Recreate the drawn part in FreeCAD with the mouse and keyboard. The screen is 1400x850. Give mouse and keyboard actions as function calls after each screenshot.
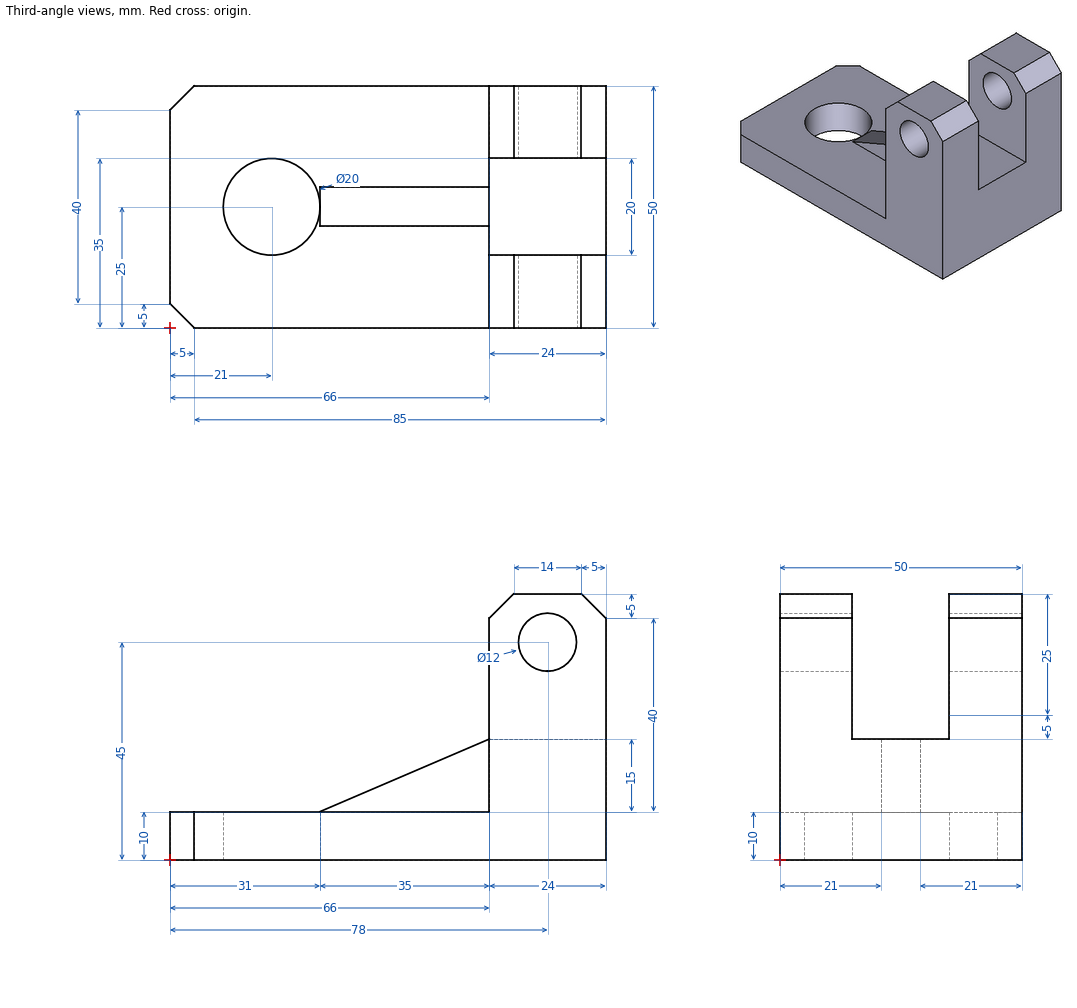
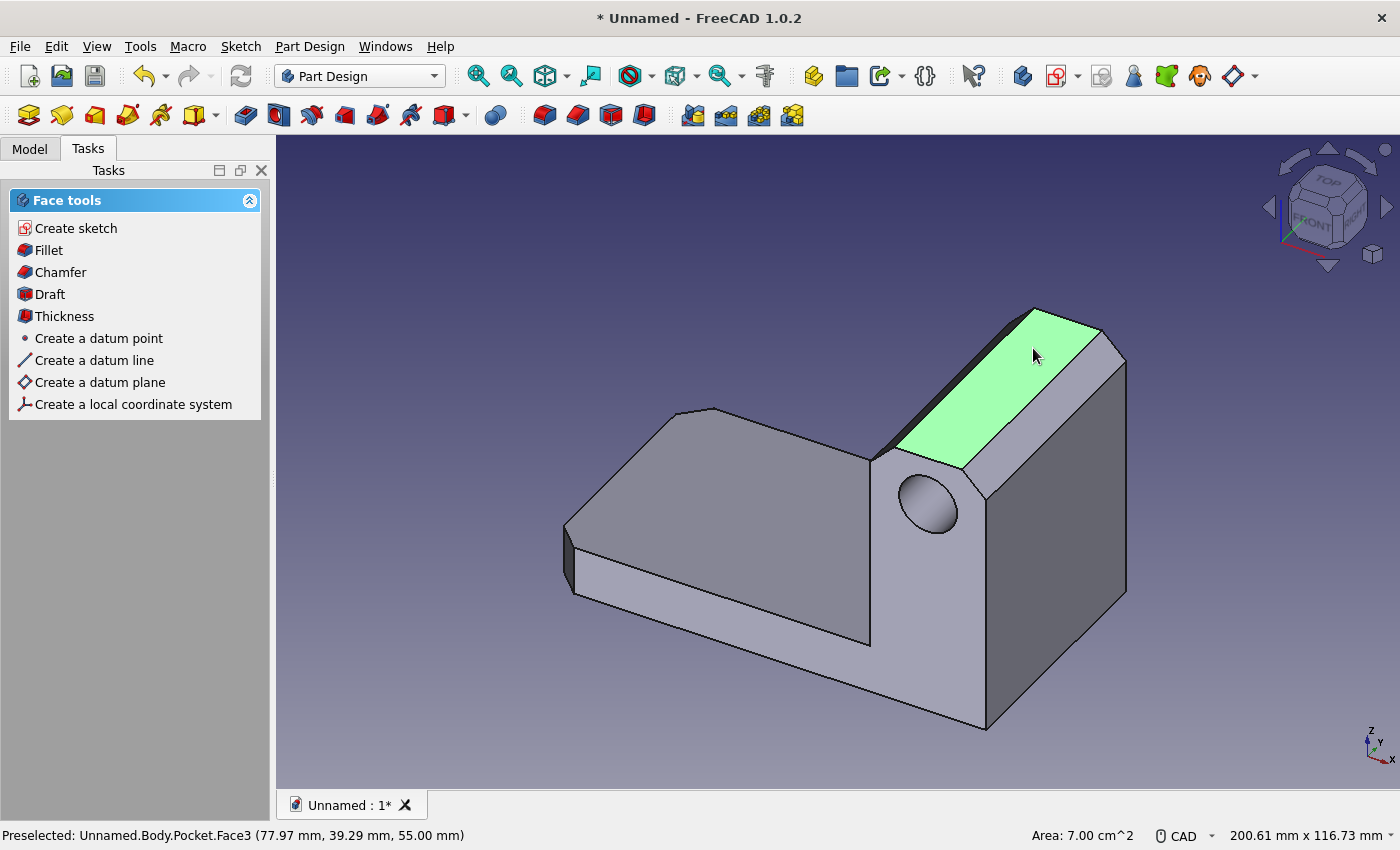
click(1056, 76)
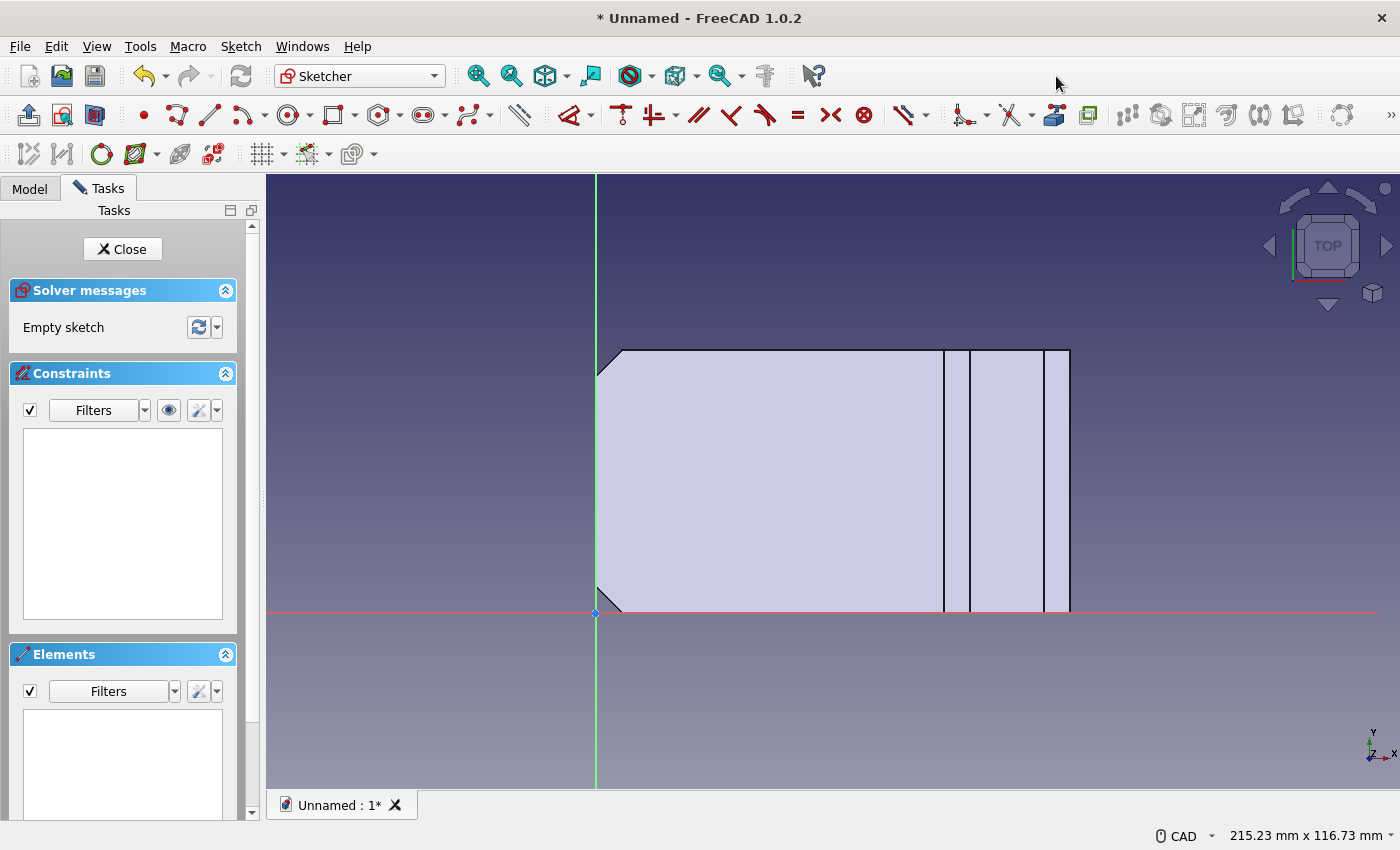
scroll(1086, 481, up, 7)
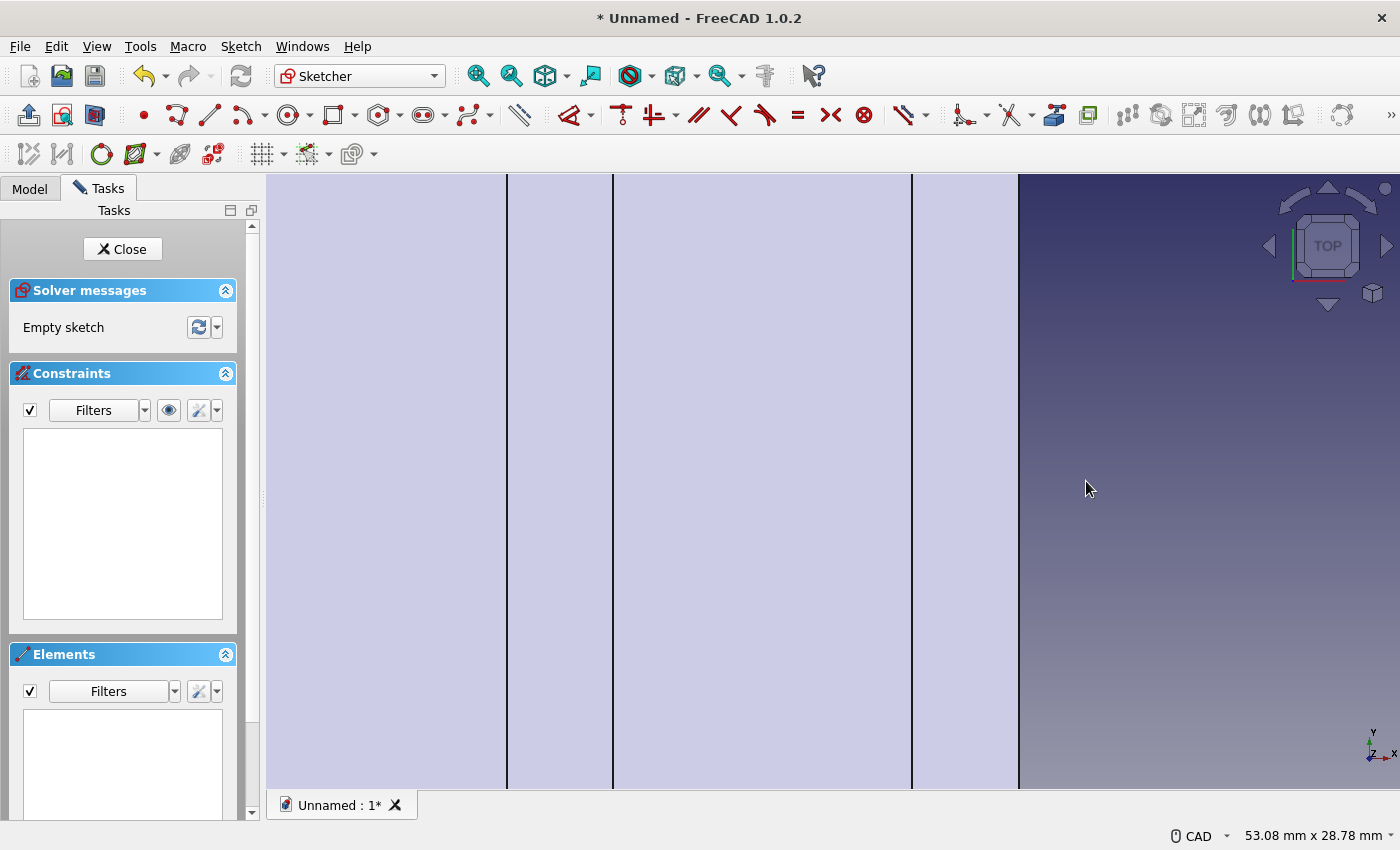
click(332, 116)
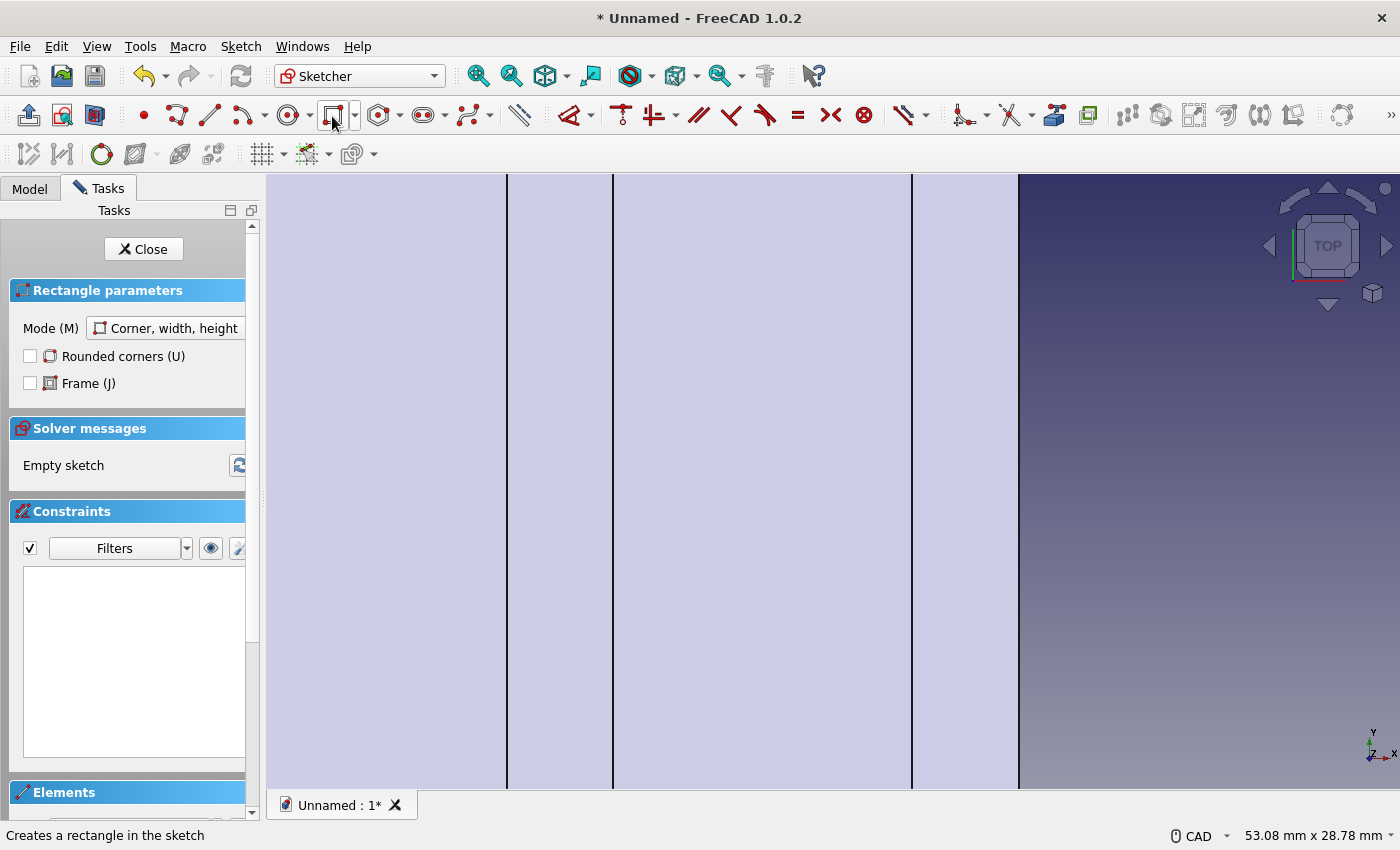
click(507, 268)
move(1019, 695)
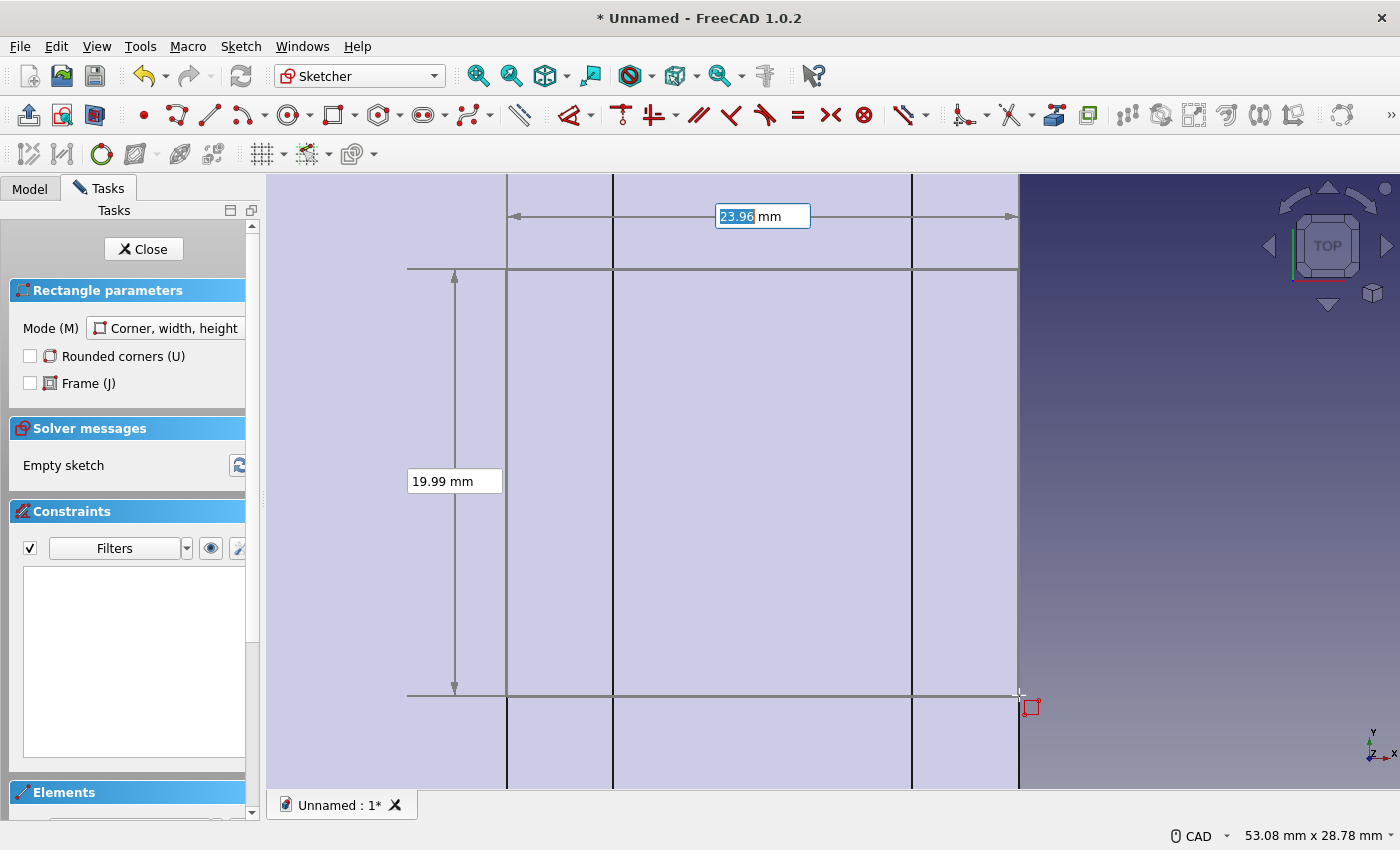
text(24)
key(Tab)
text(20)
key(Return)
key(Escape)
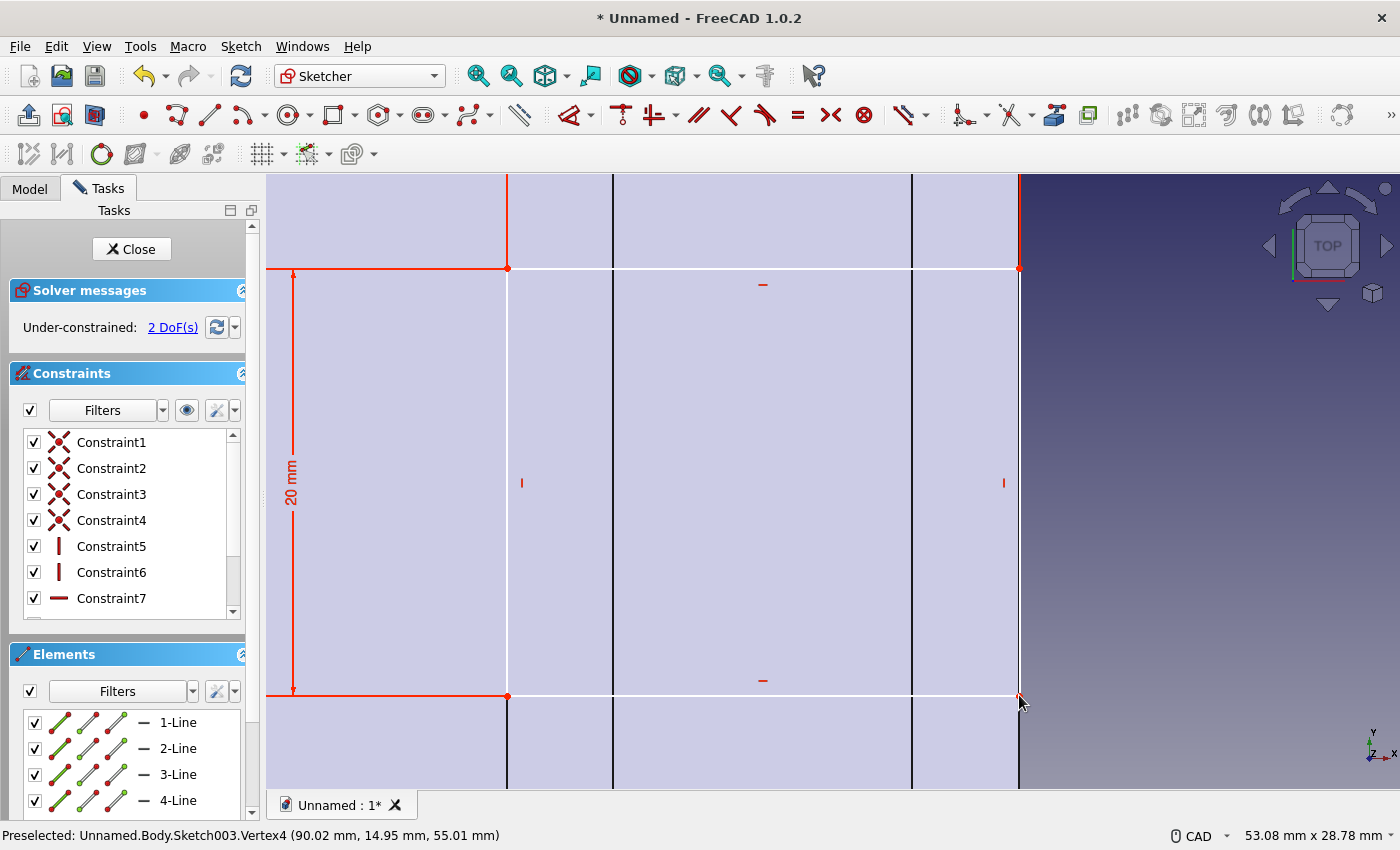
click(568, 116)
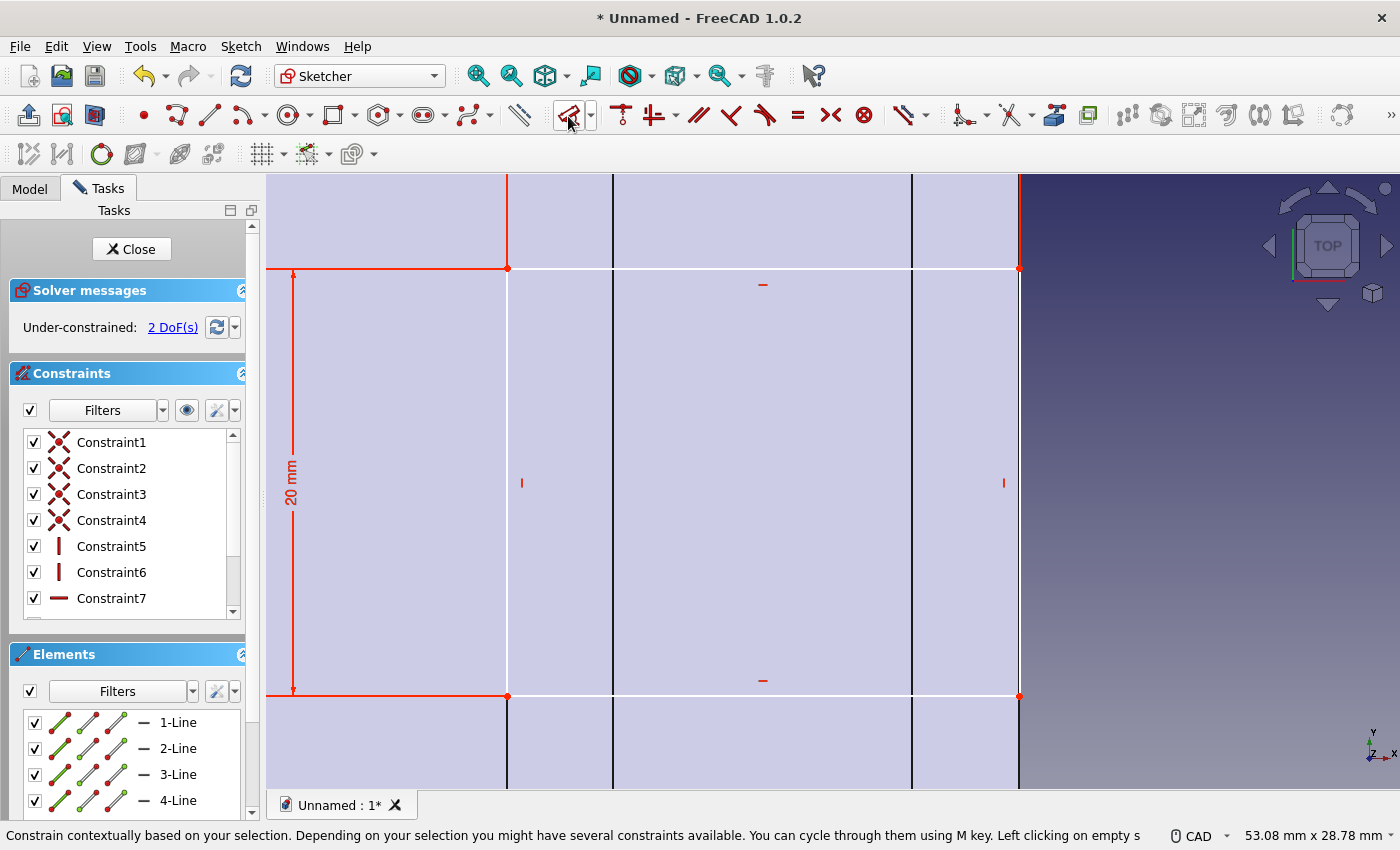
click(507, 269)
click(400, 235)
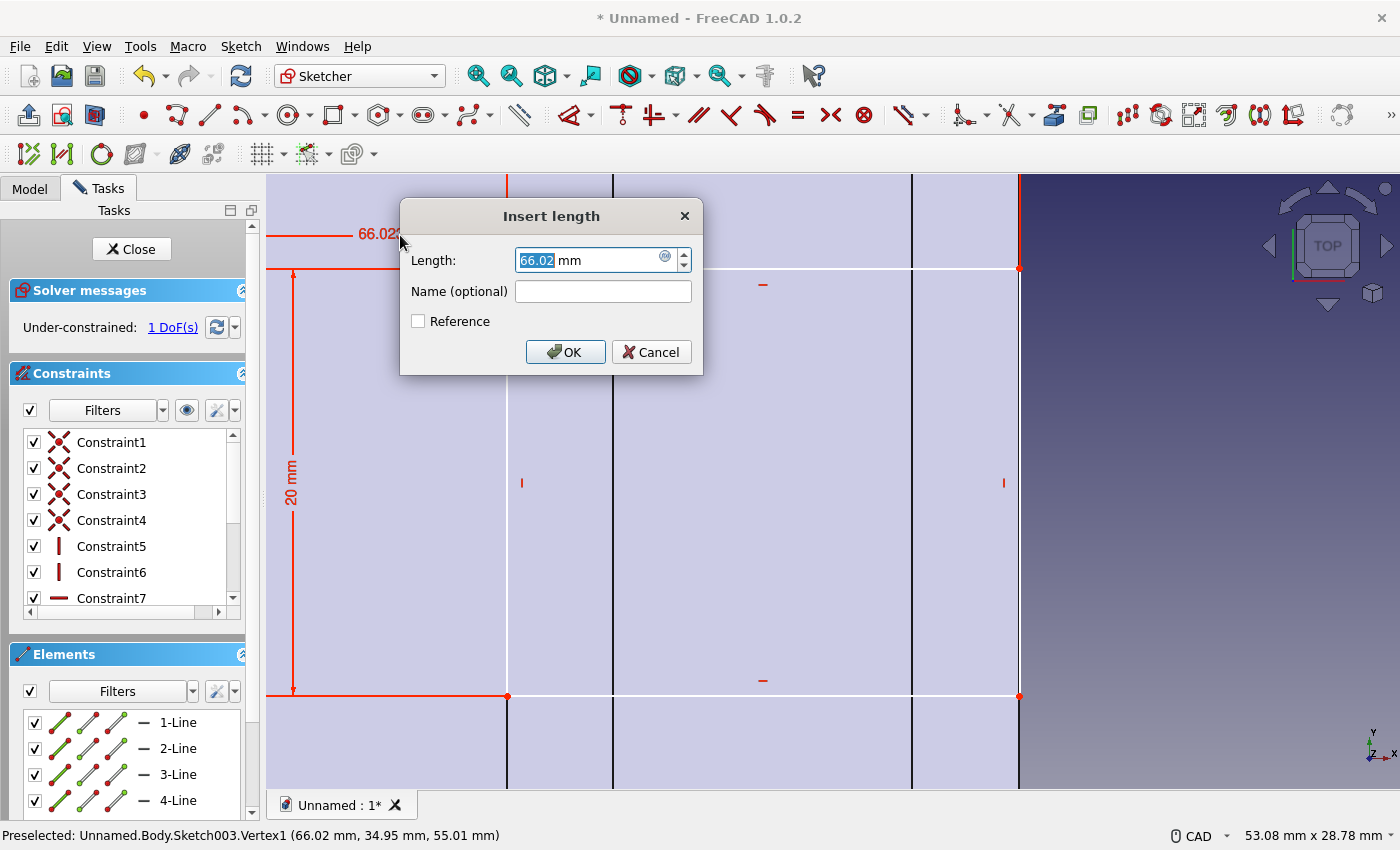
text(66)
key(Return)